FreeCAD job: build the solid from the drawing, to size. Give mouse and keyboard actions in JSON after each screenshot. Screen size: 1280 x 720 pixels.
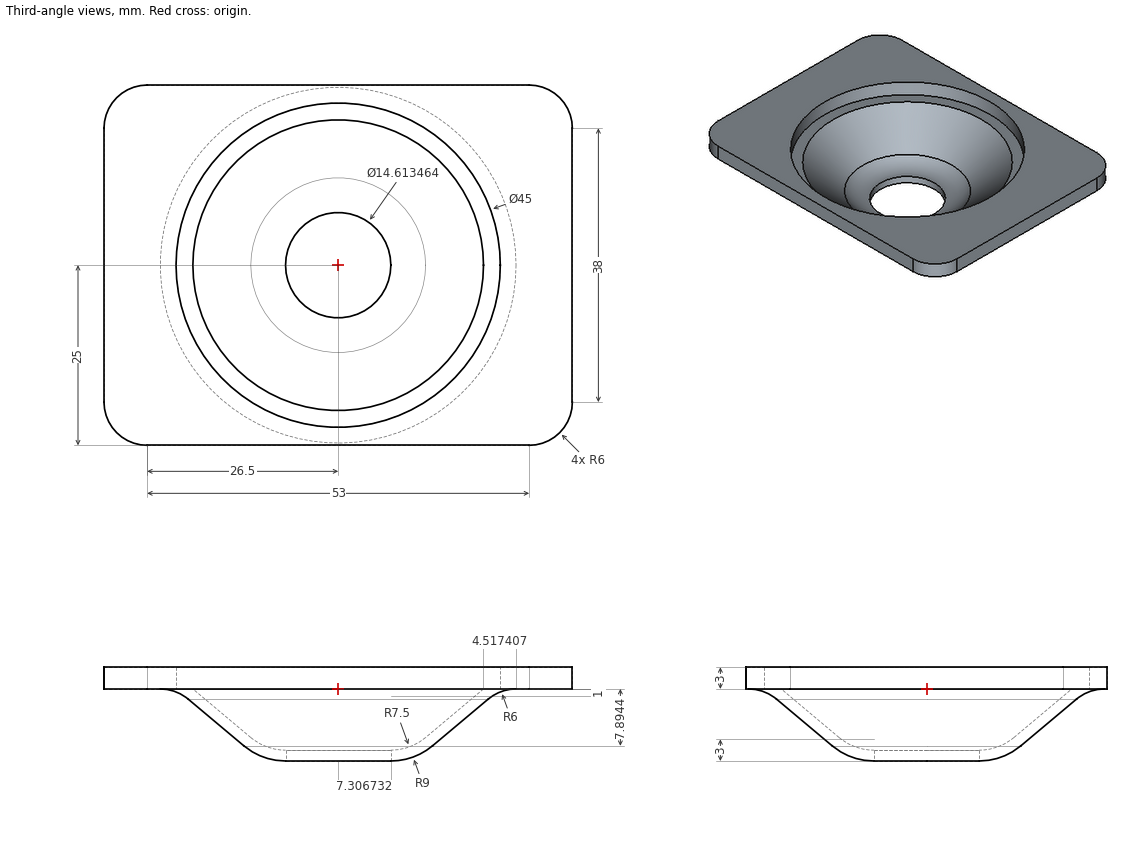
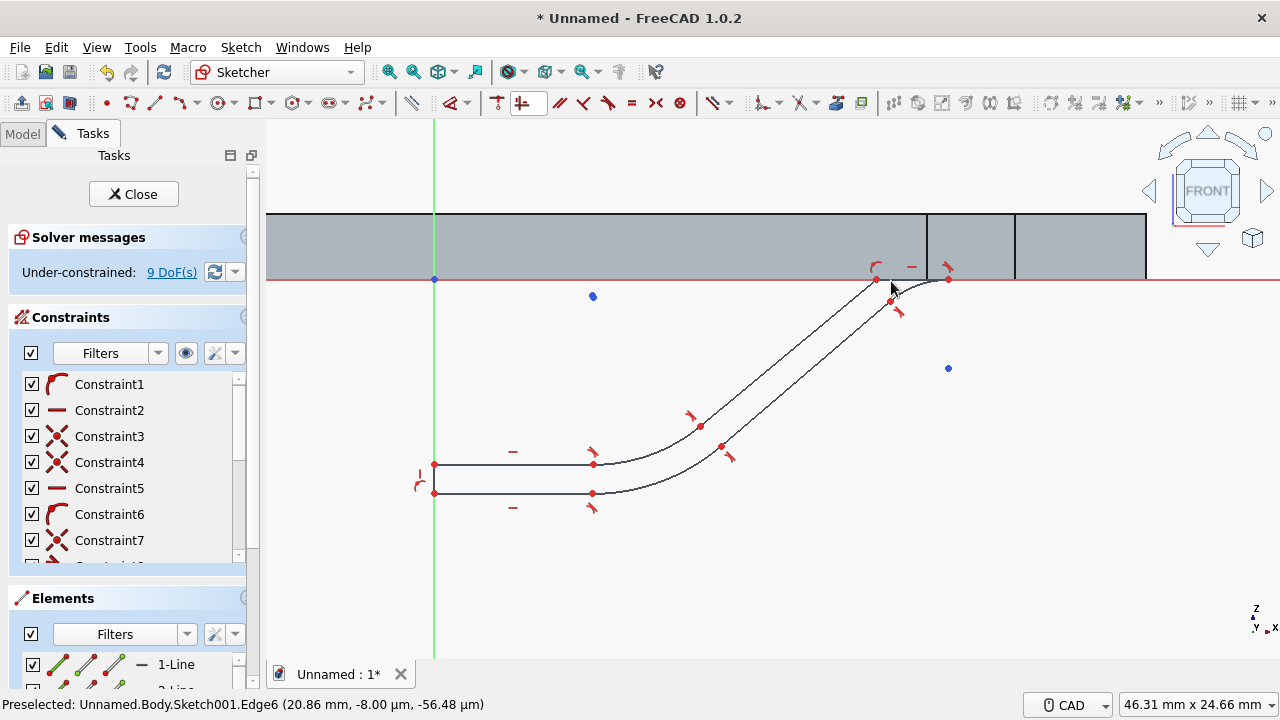
{"action": "left_click", "coordinate": [634, 489]}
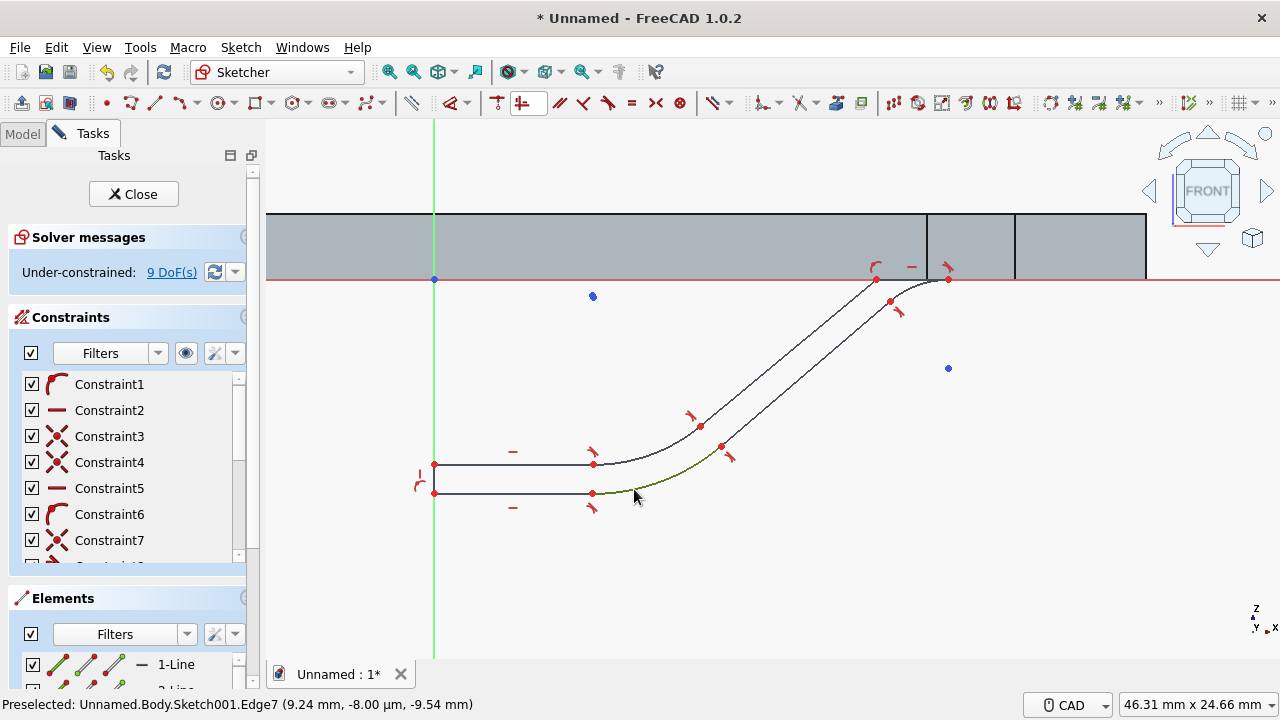
{"action": "left_click", "coordinate": [628, 461]}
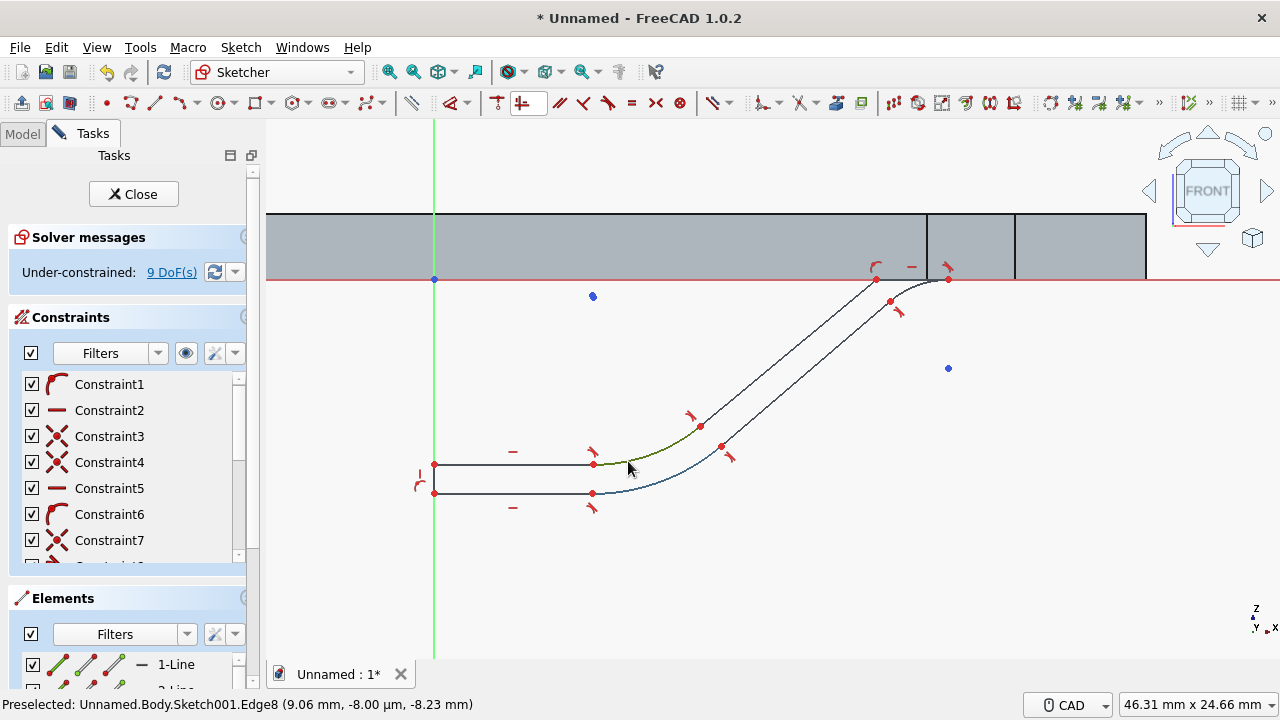
{"action": "left_click", "coordinate": [498, 104]}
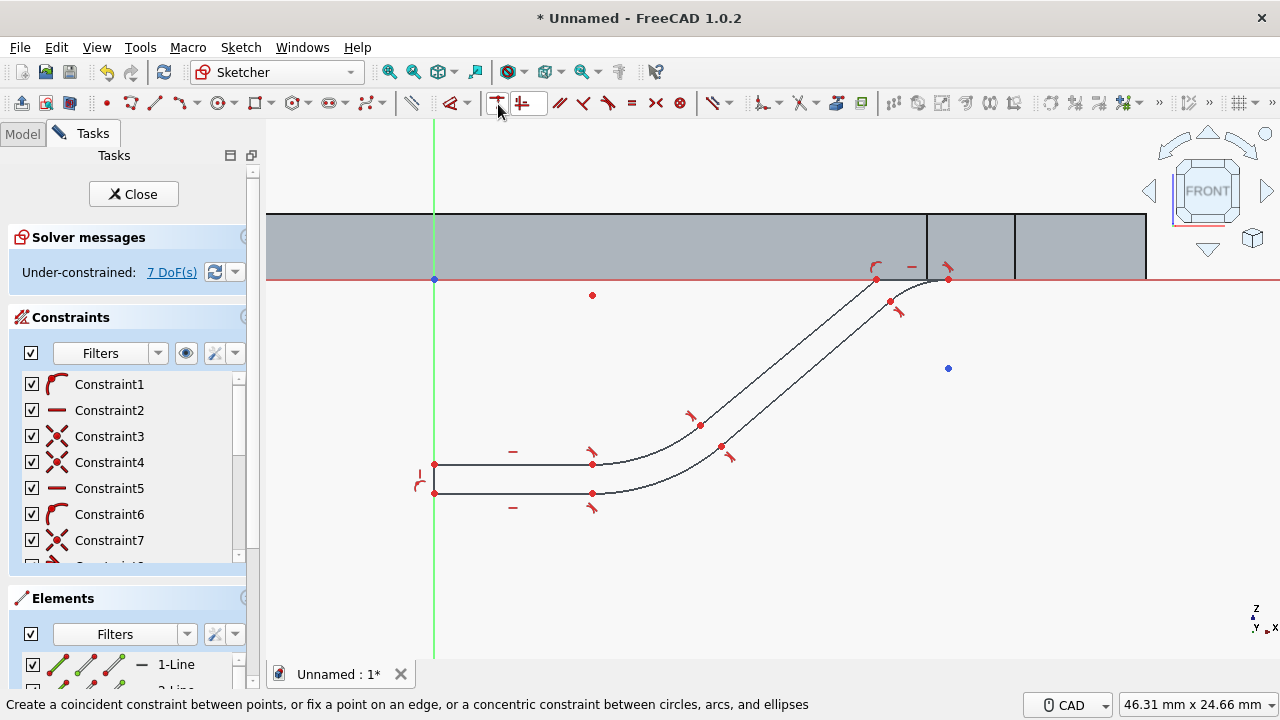
{"action": "left_click", "coordinate": [450, 104]}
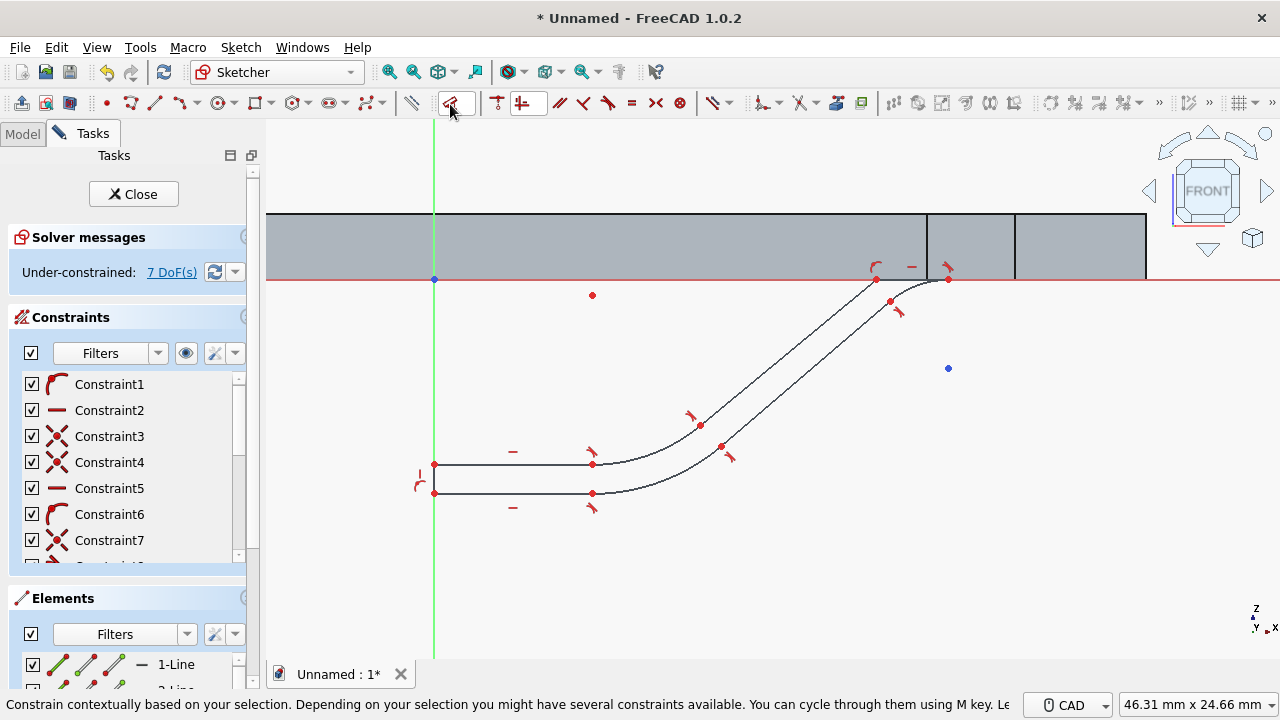
{"action": "left_click", "coordinate": [634, 489]}
{"action": "left_click", "coordinate": [641, 520]}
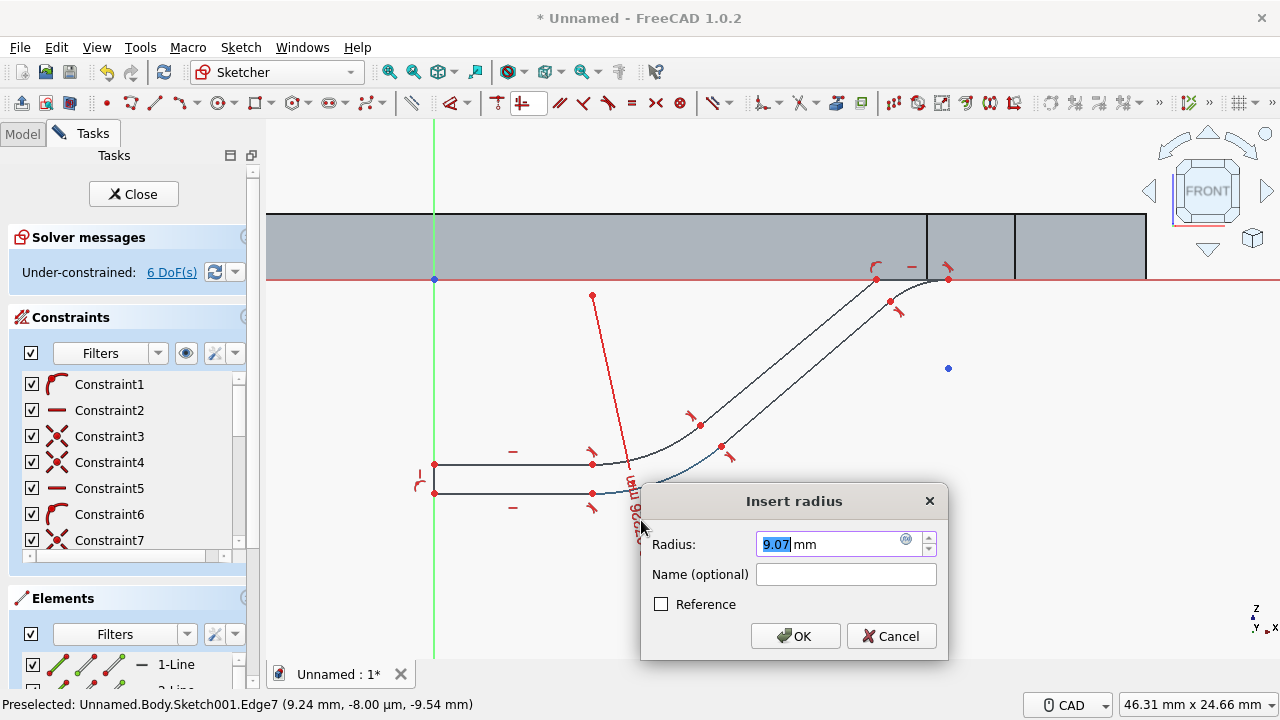
{"action": "type", "text": "9"}
{"action": "key", "text": "Return"}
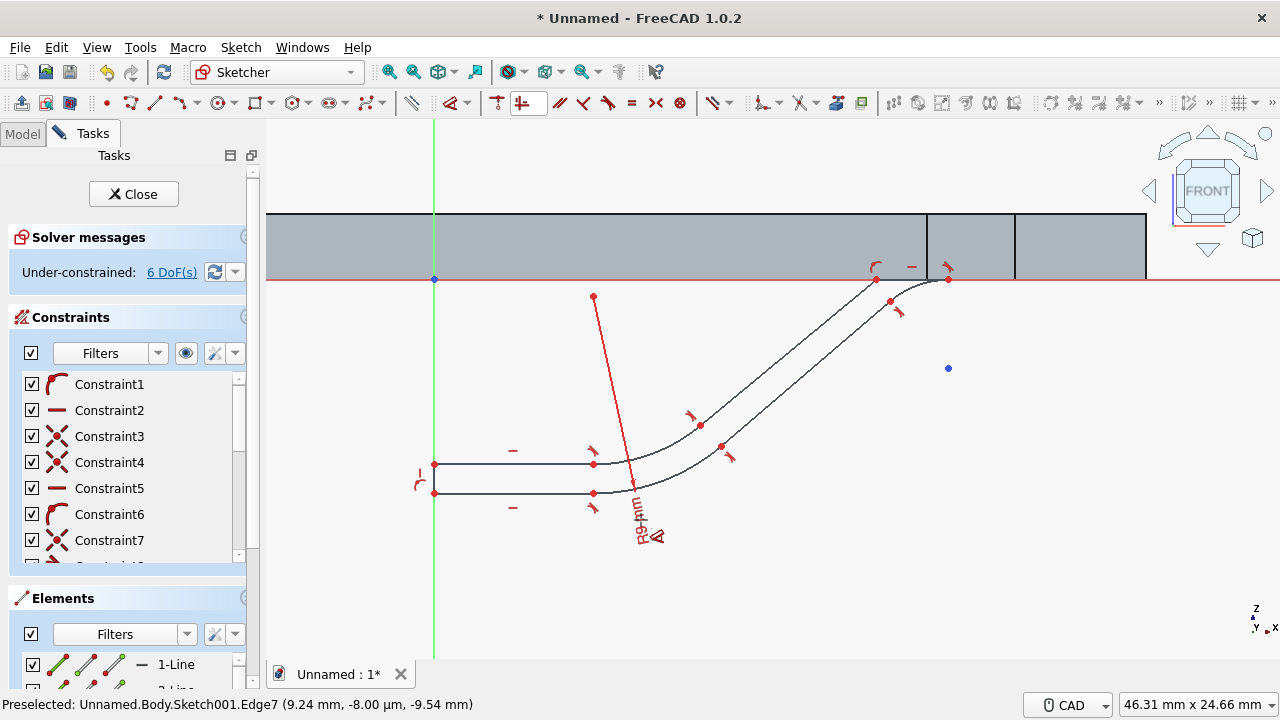
{"action": "left_click", "coordinate": [628, 461]}
{"action": "left_click", "coordinate": [451, 437]}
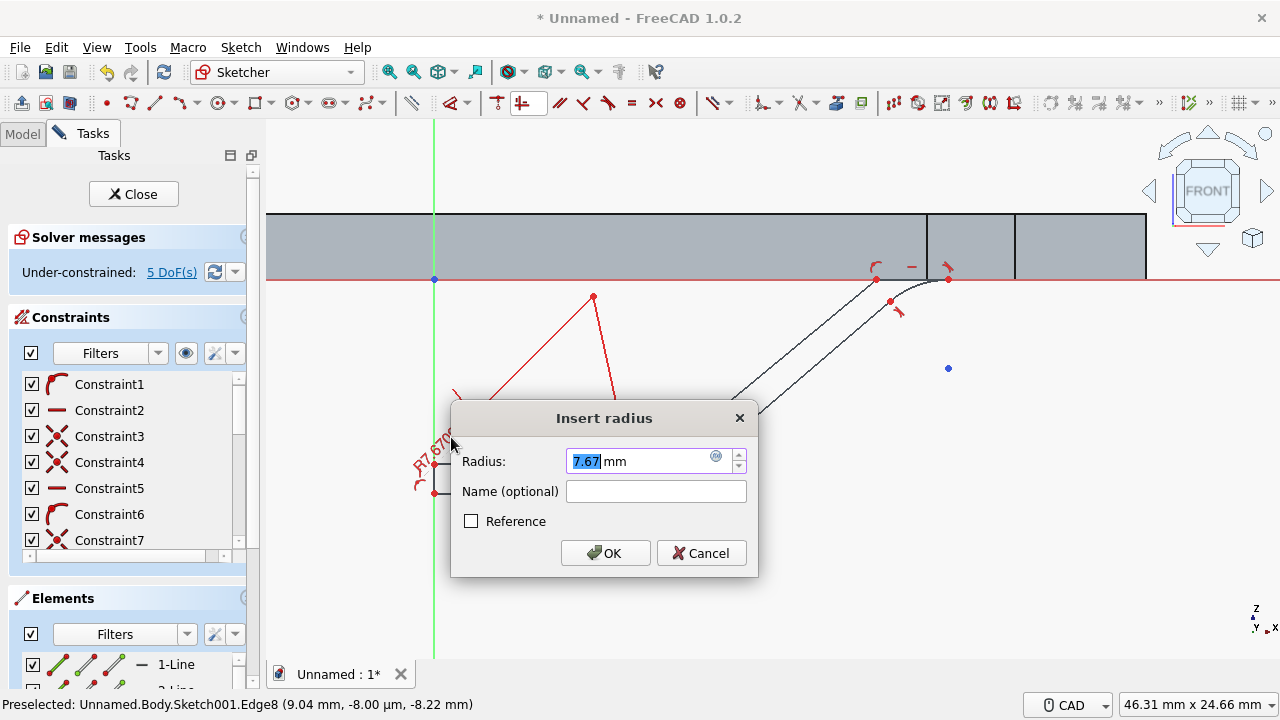
{"action": "type", "text": "7.5"}
{"action": "key", "text": "Return"}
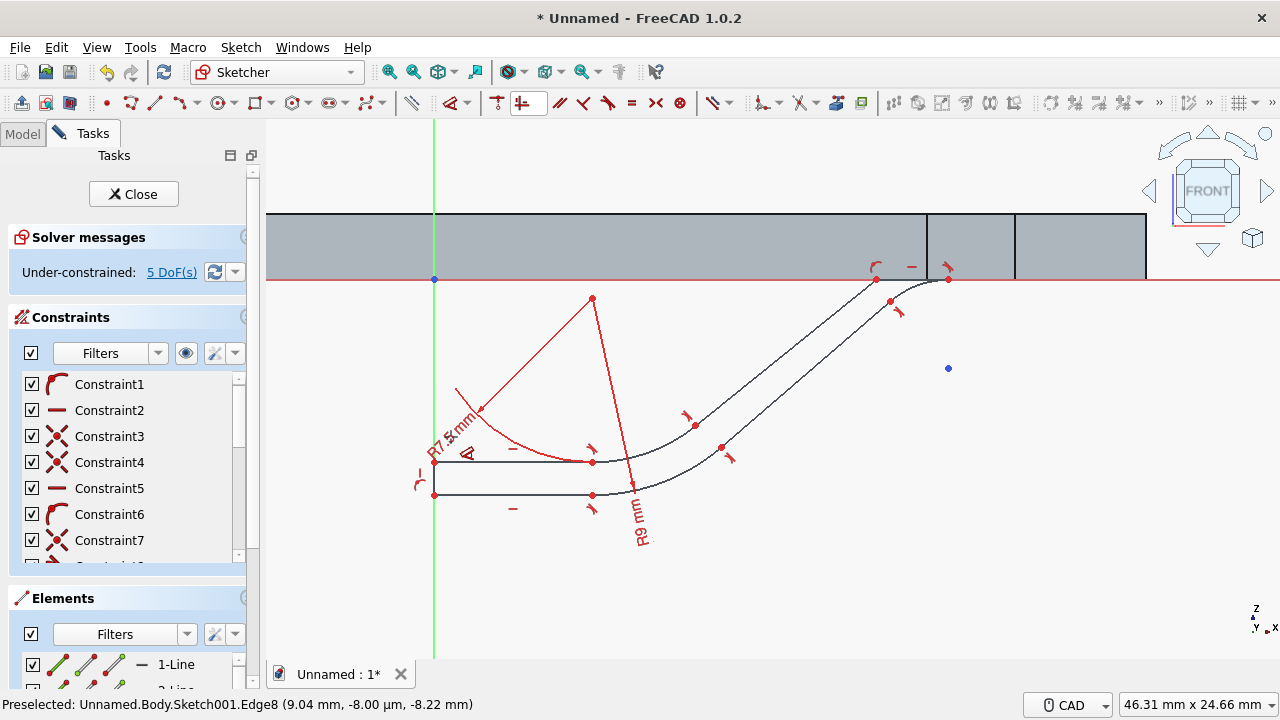
{"action": "scroll", "coordinate": [906, 291], "scroll_direction": "up", "scroll_amount": 2}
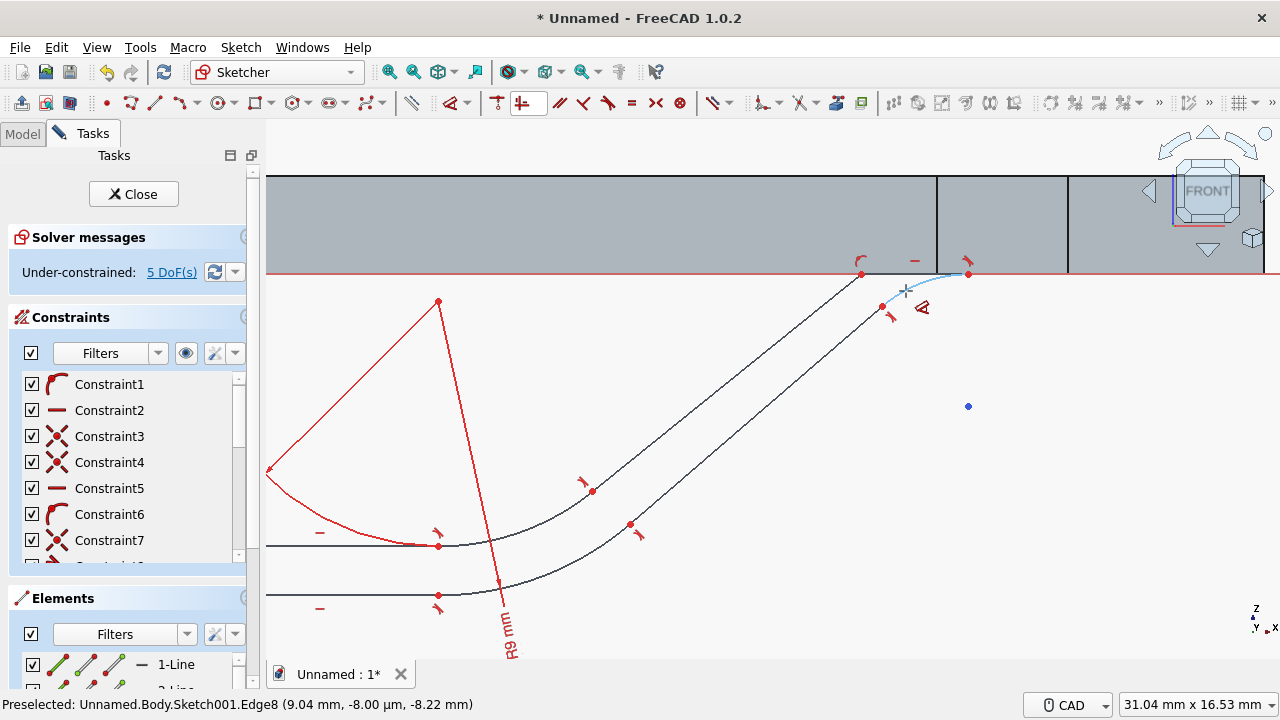
{"action": "left_click", "coordinate": [906, 290]}
{"action": "left_click", "coordinate": [970, 242]}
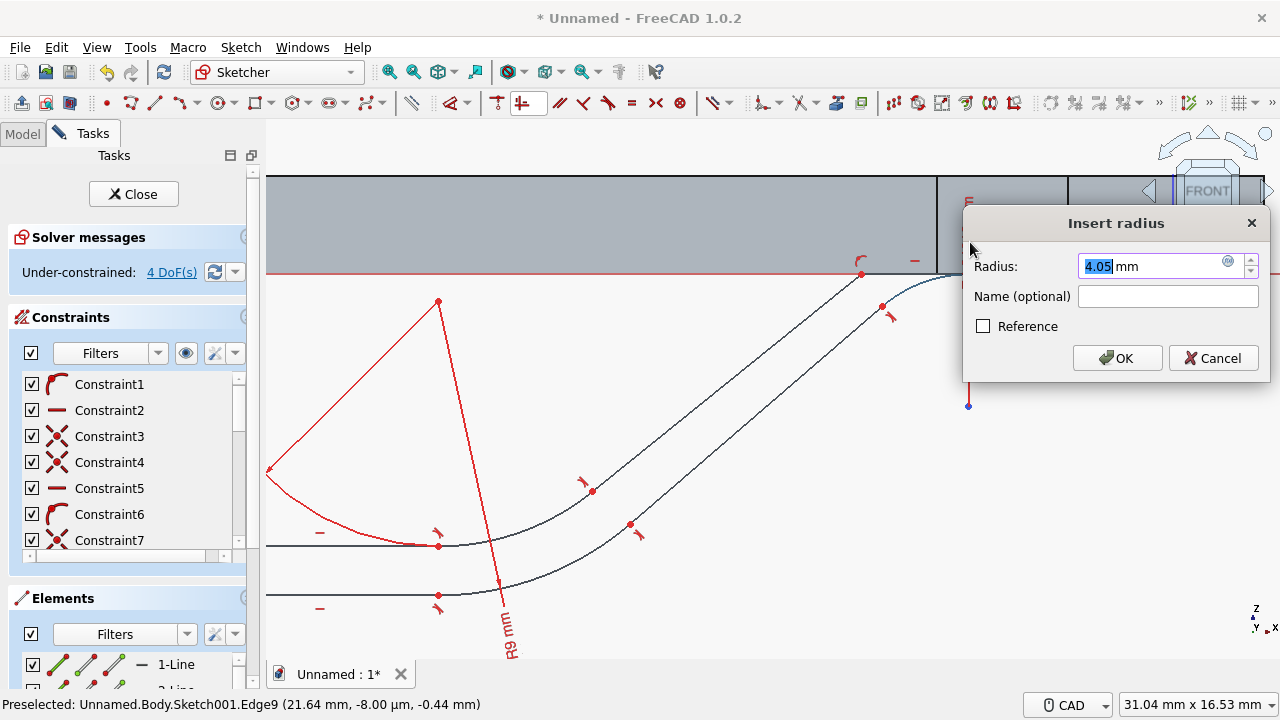
{"action": "type", "text": "6"}
{"action": "key", "text": "Return"}